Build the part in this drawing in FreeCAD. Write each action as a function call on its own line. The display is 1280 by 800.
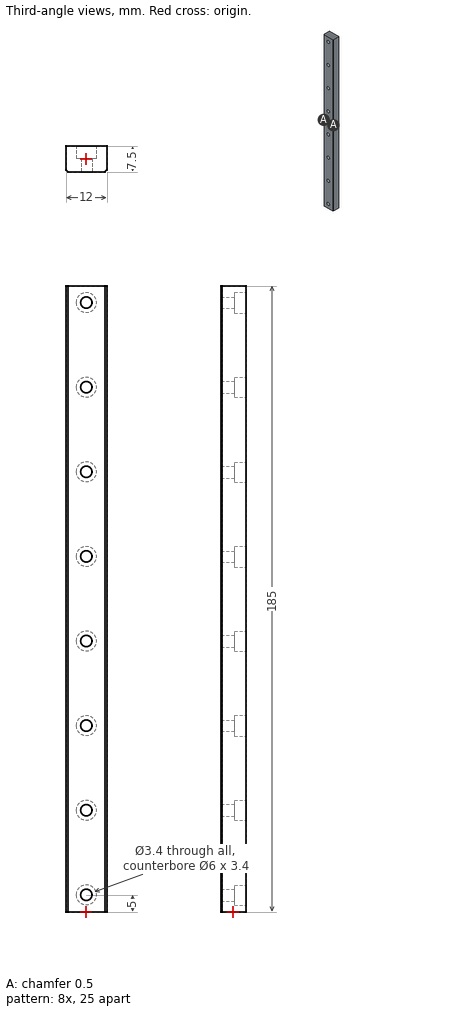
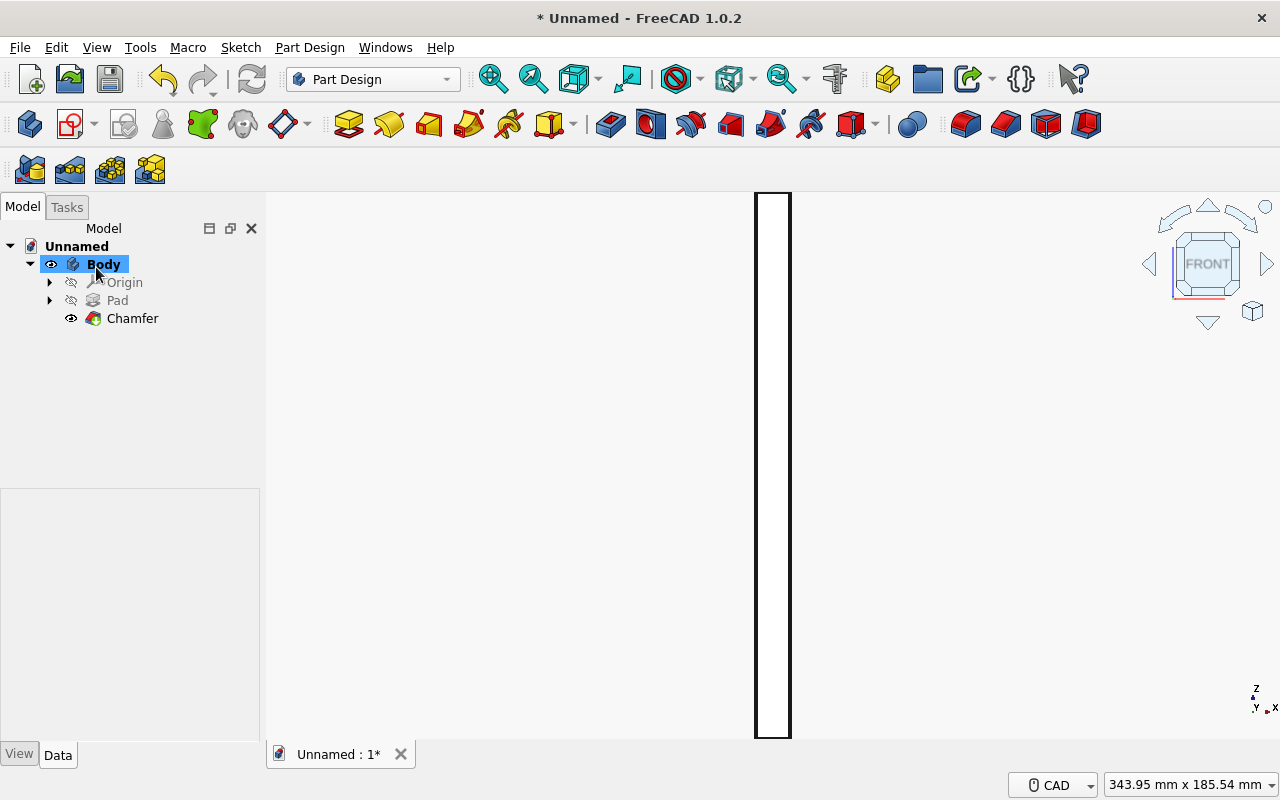
click(773, 231)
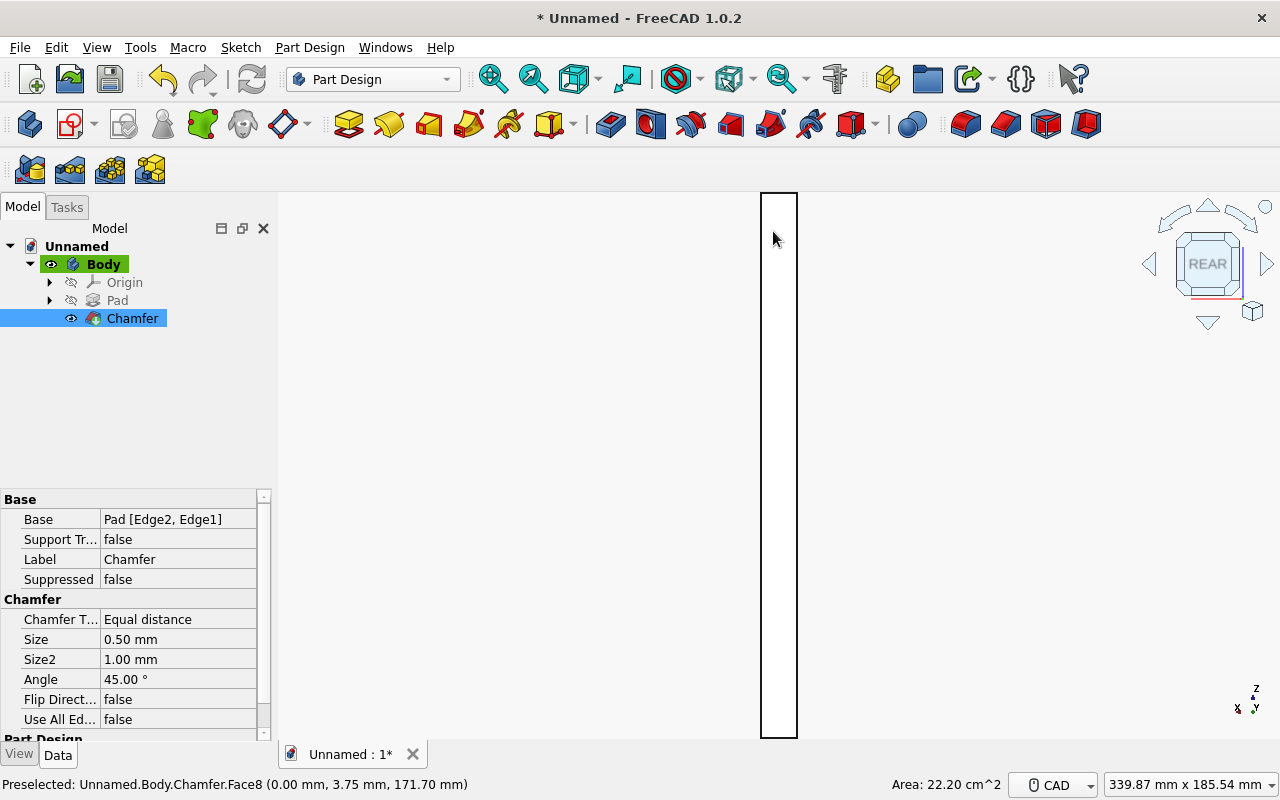
click(70, 124)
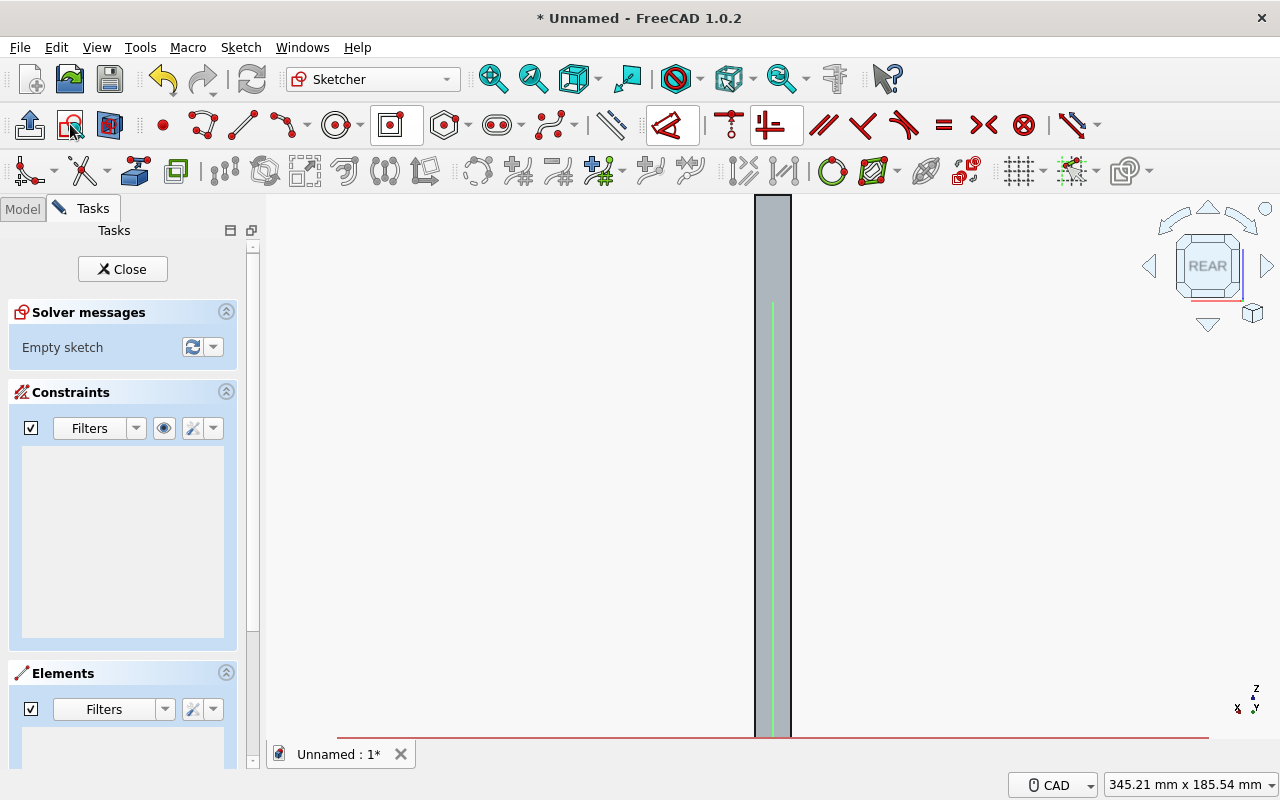
scroll(704, 466, down, 5)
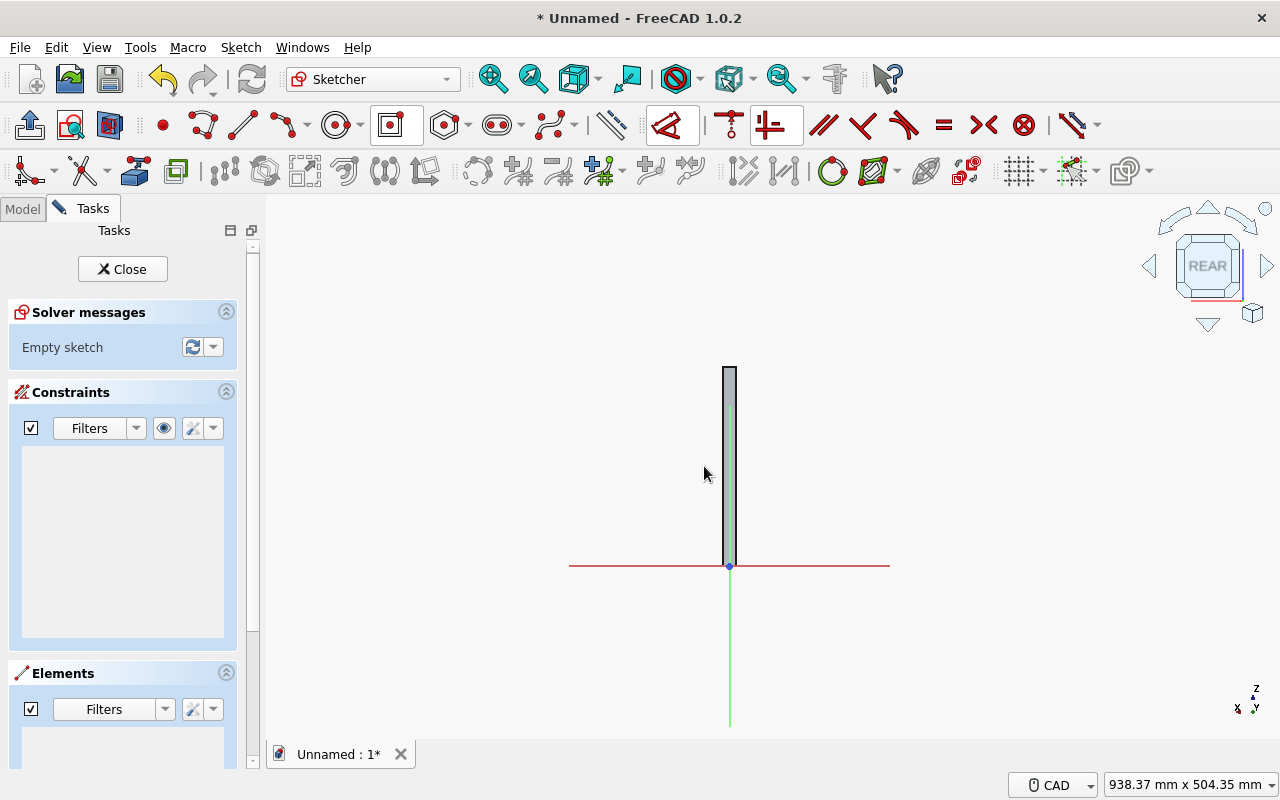
scroll(731, 568, up, 15)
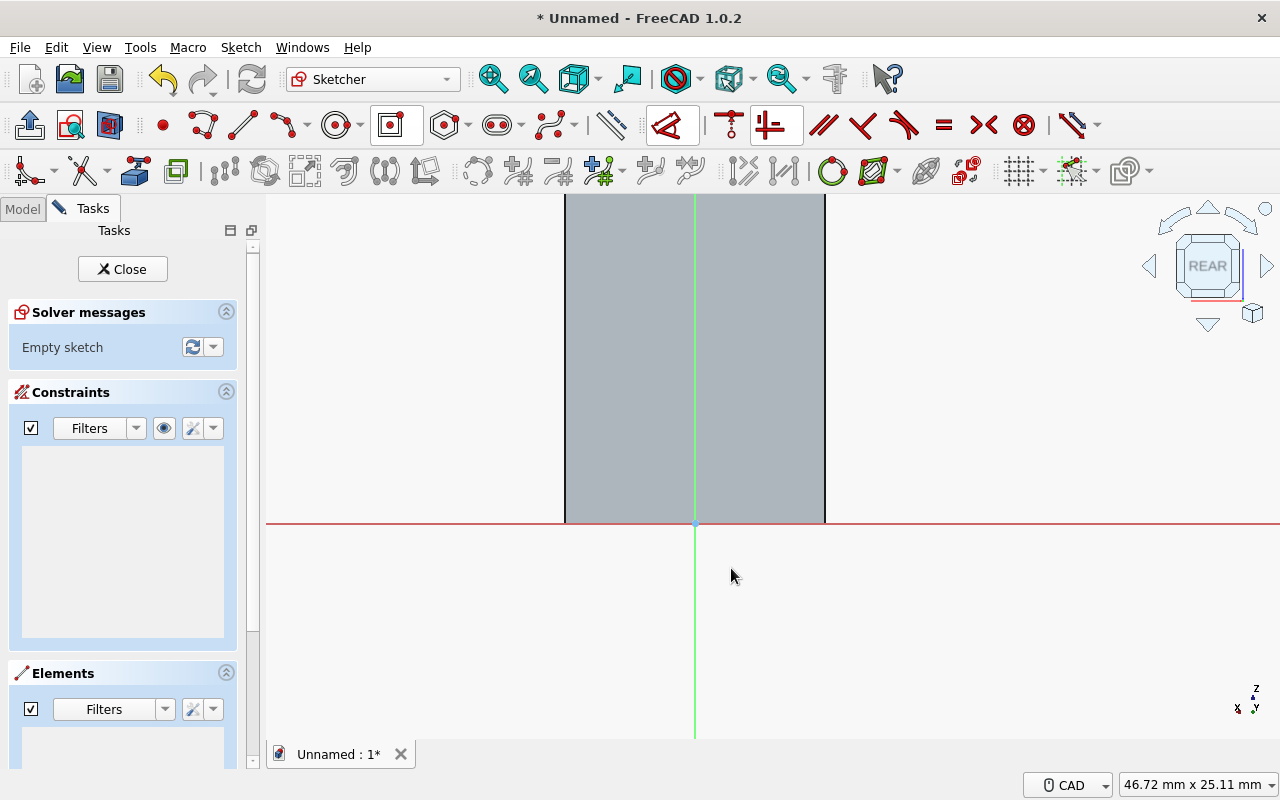
scroll(688, 439, up, 4)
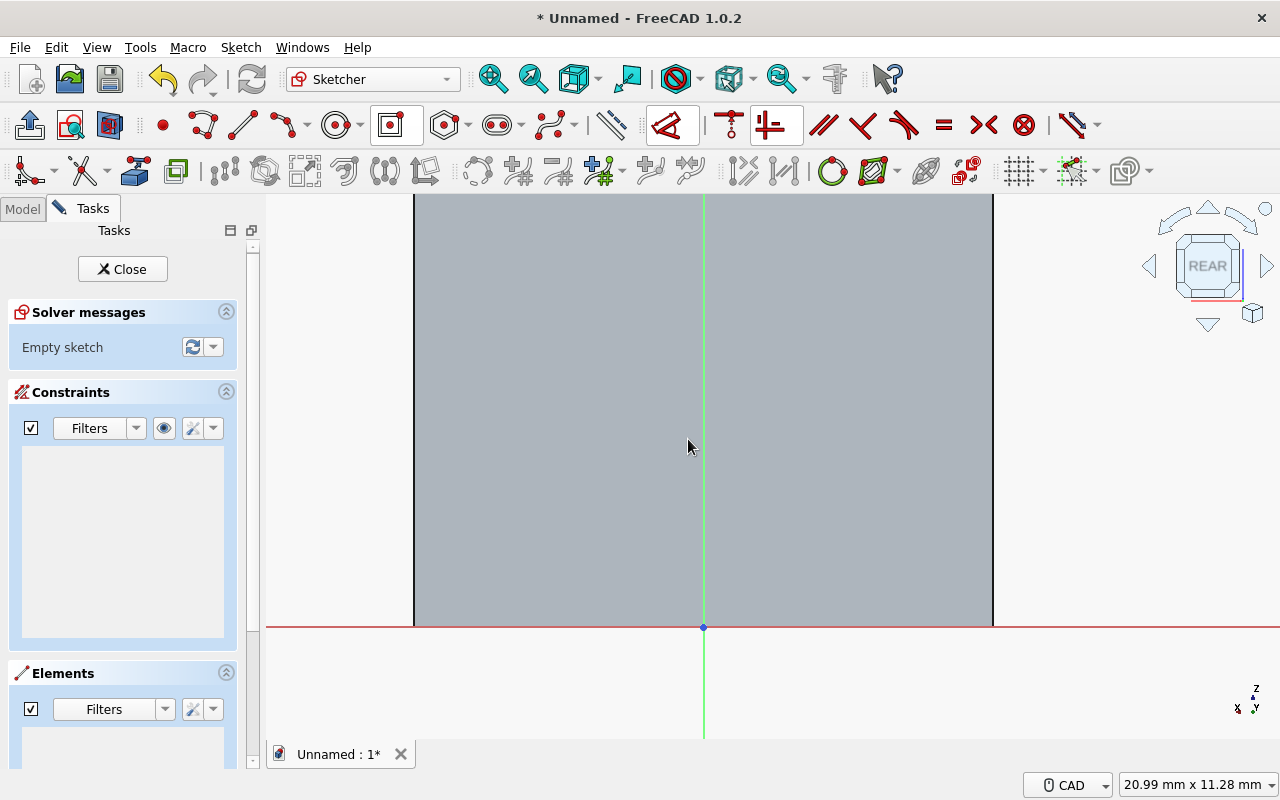
click(336, 126)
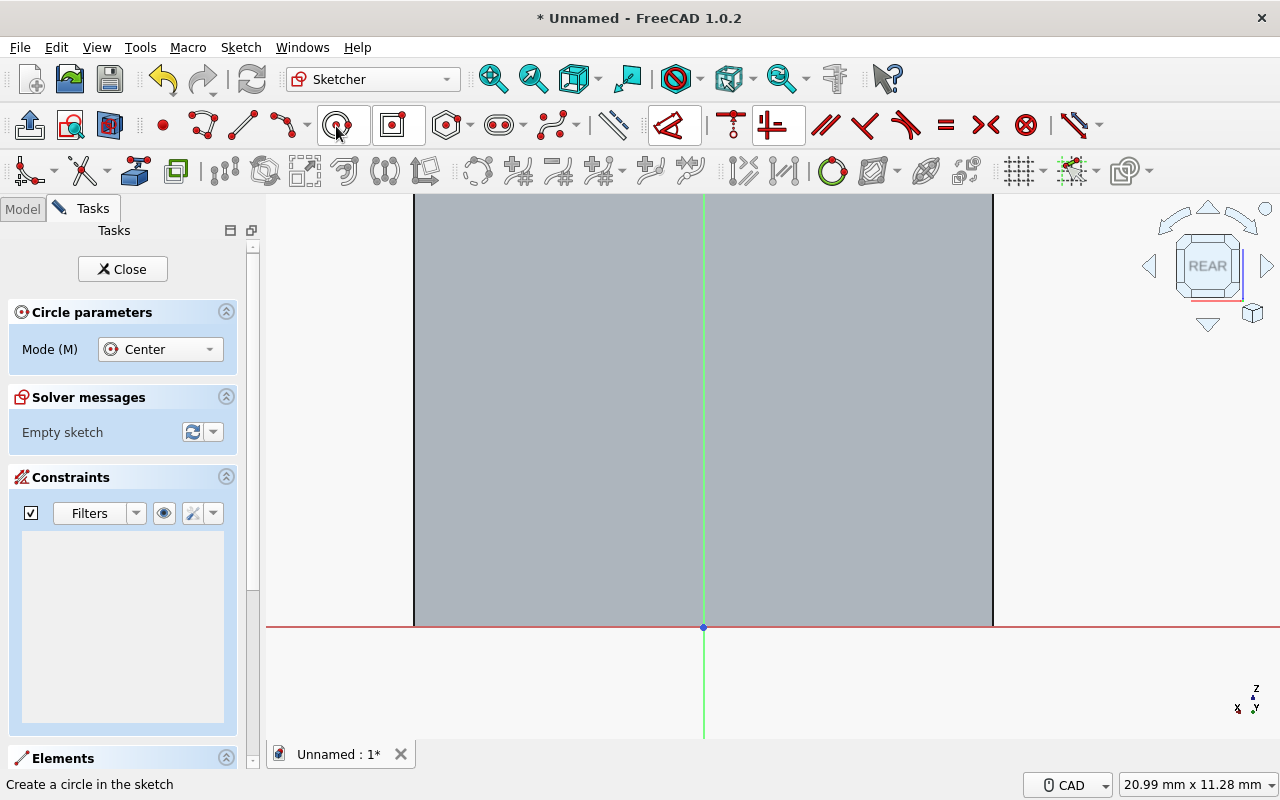
click(704, 386)
click(762, 328)
key(Escape)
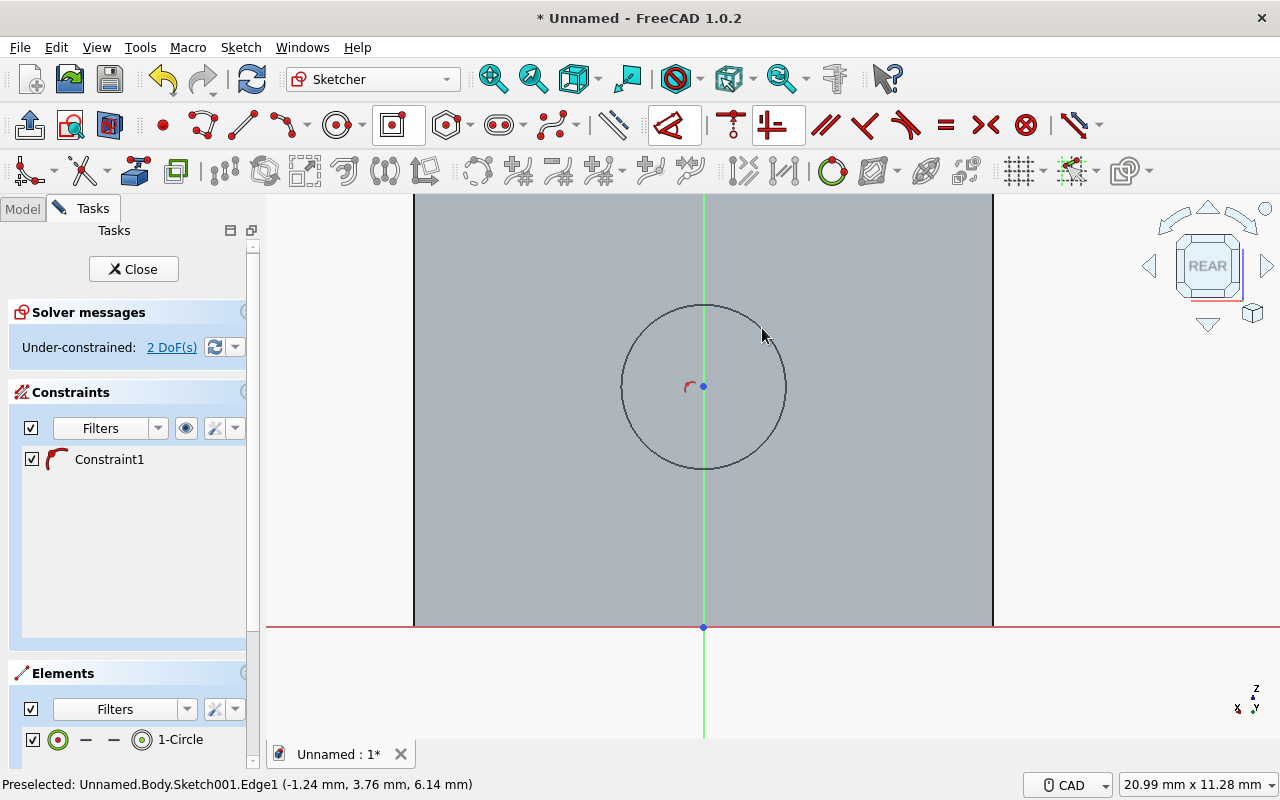
click(762, 329)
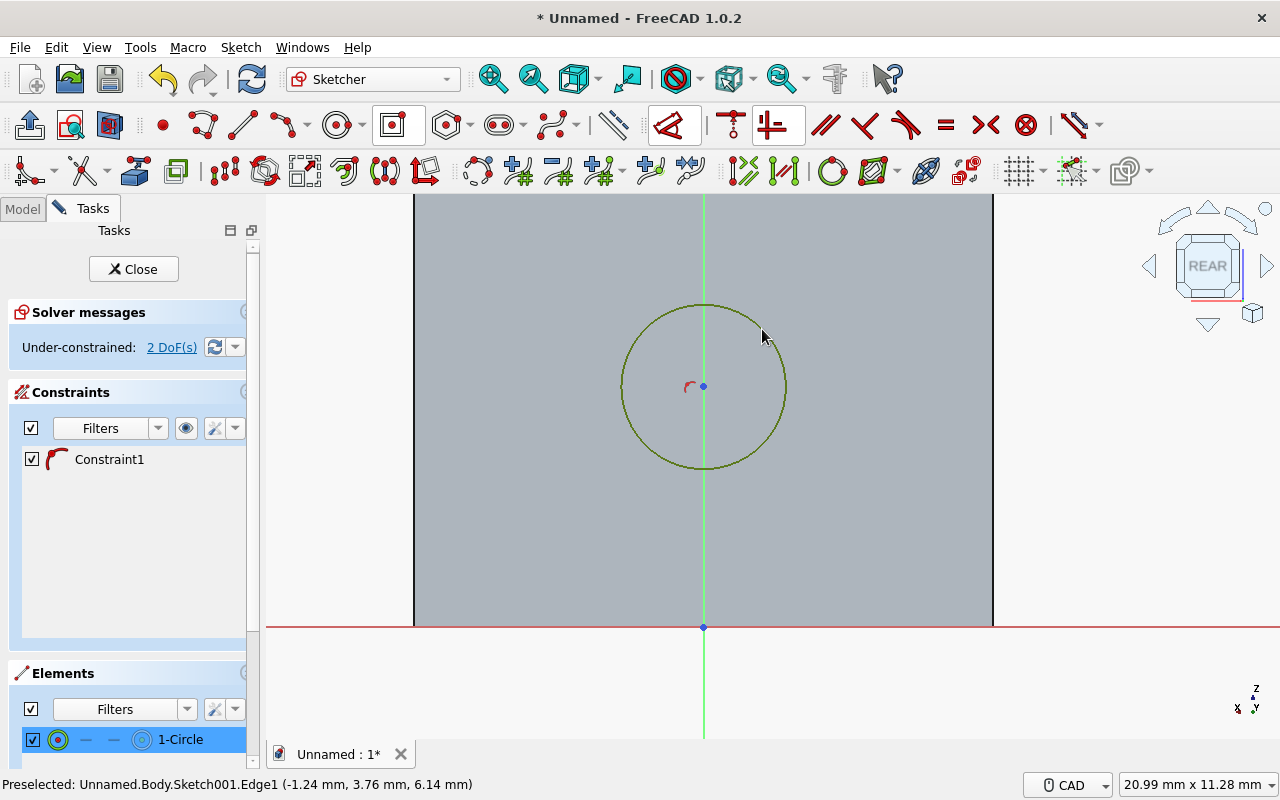
click(696, 126)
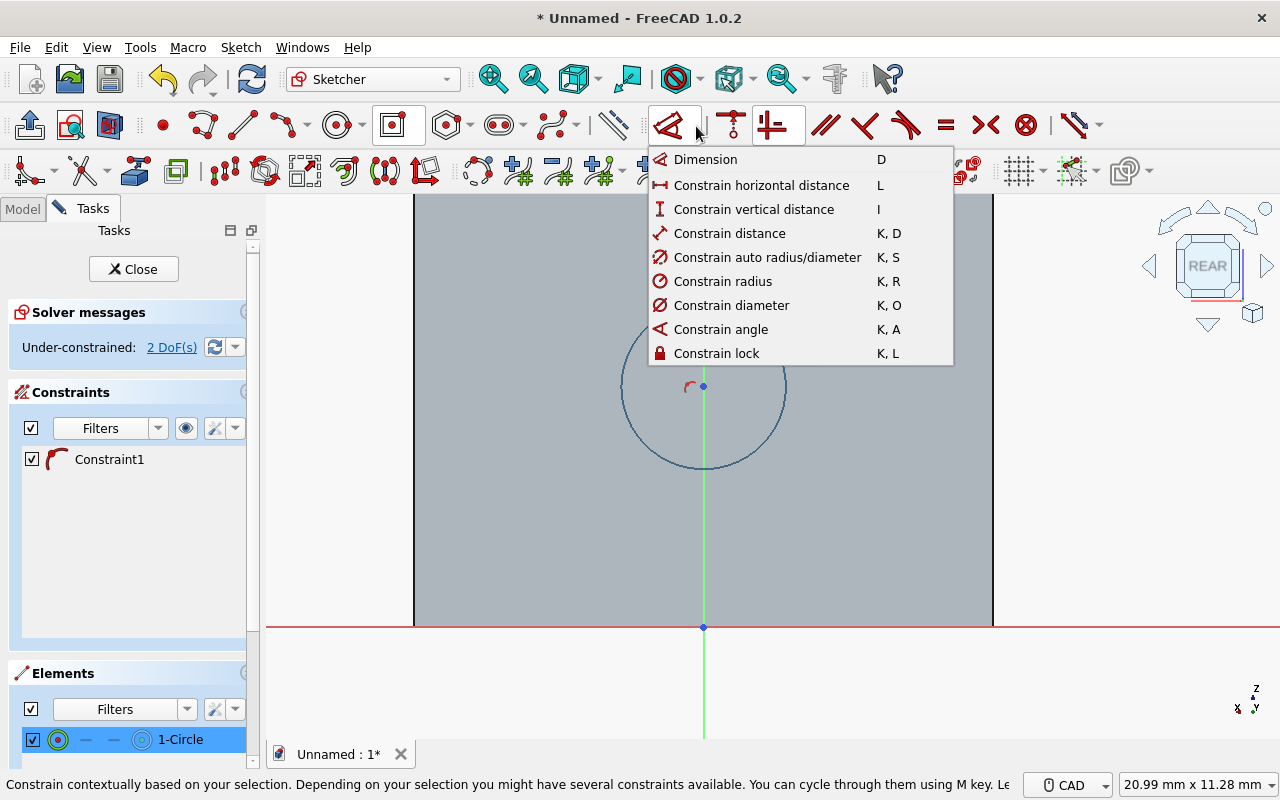
click(801, 305)